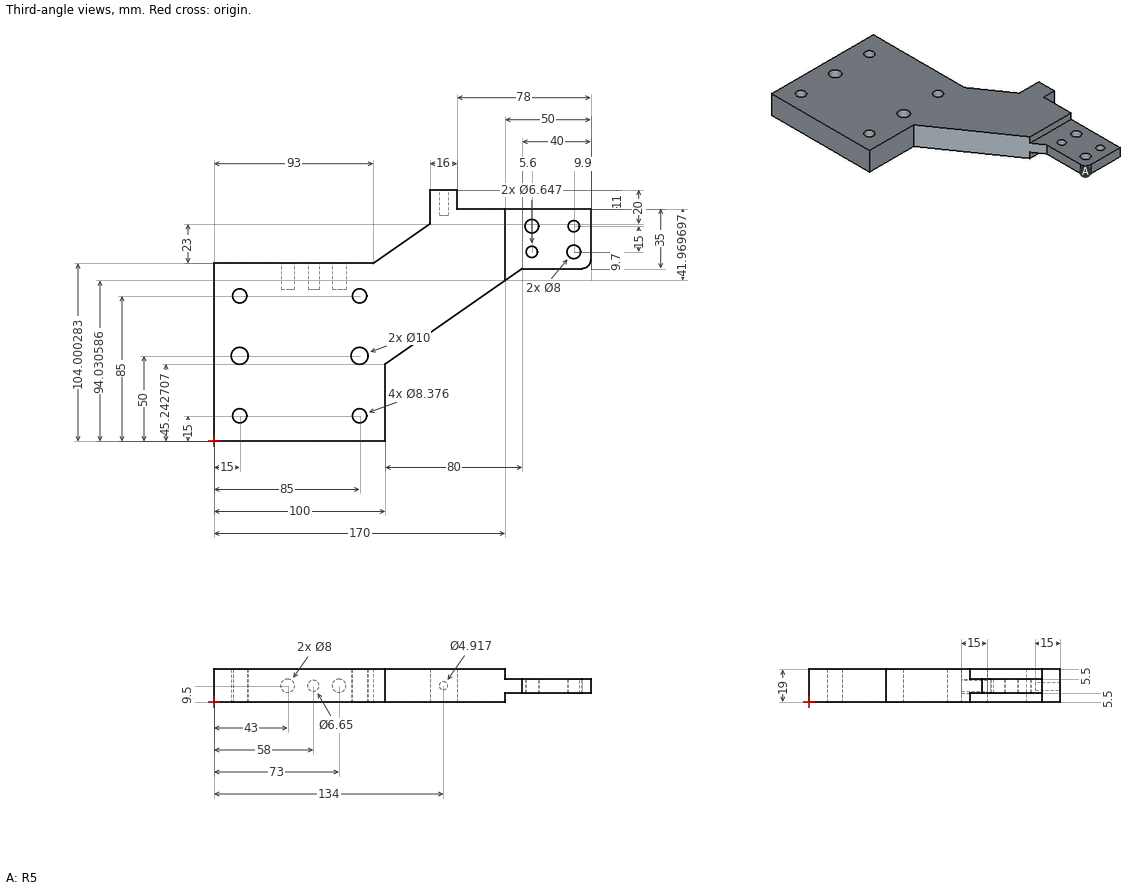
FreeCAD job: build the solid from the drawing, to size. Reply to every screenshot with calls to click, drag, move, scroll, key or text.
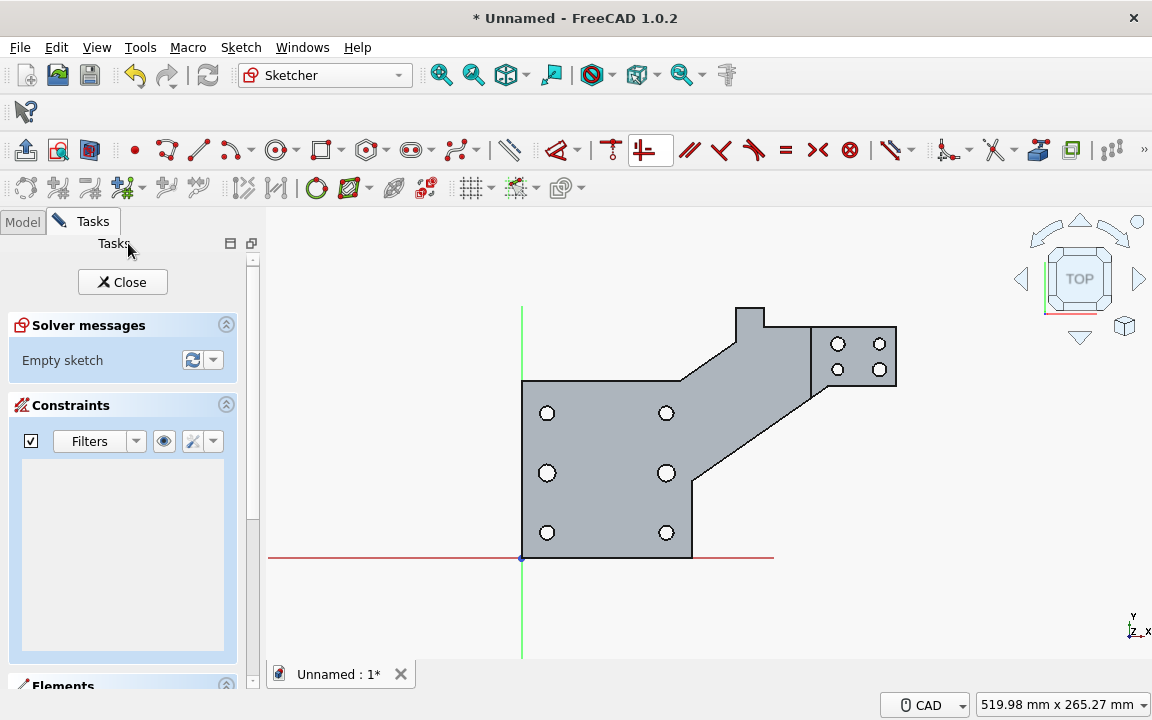
click(90, 150)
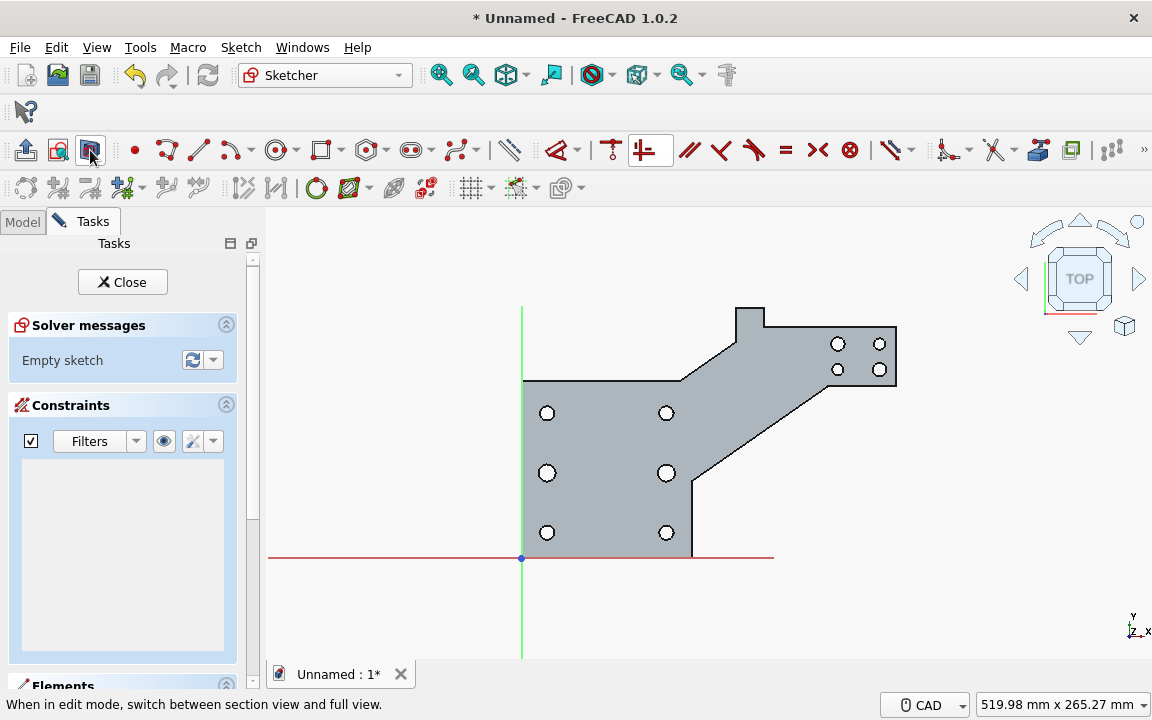
scroll(924, 339, up, 7)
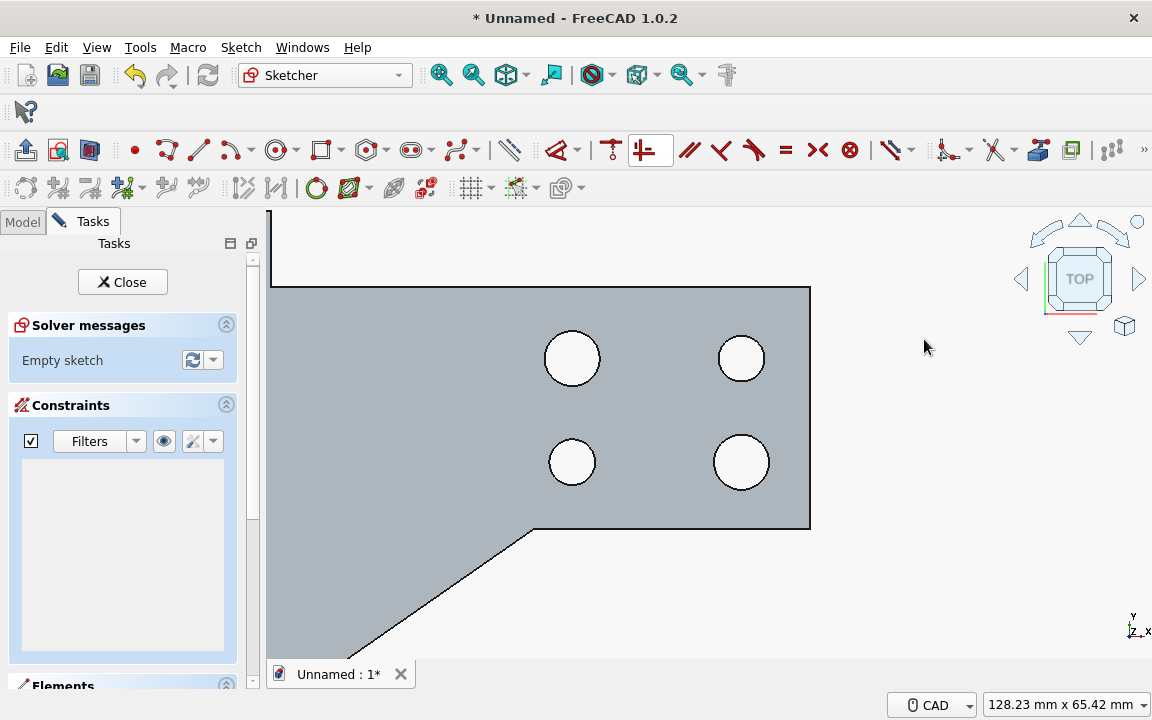
click(322, 150)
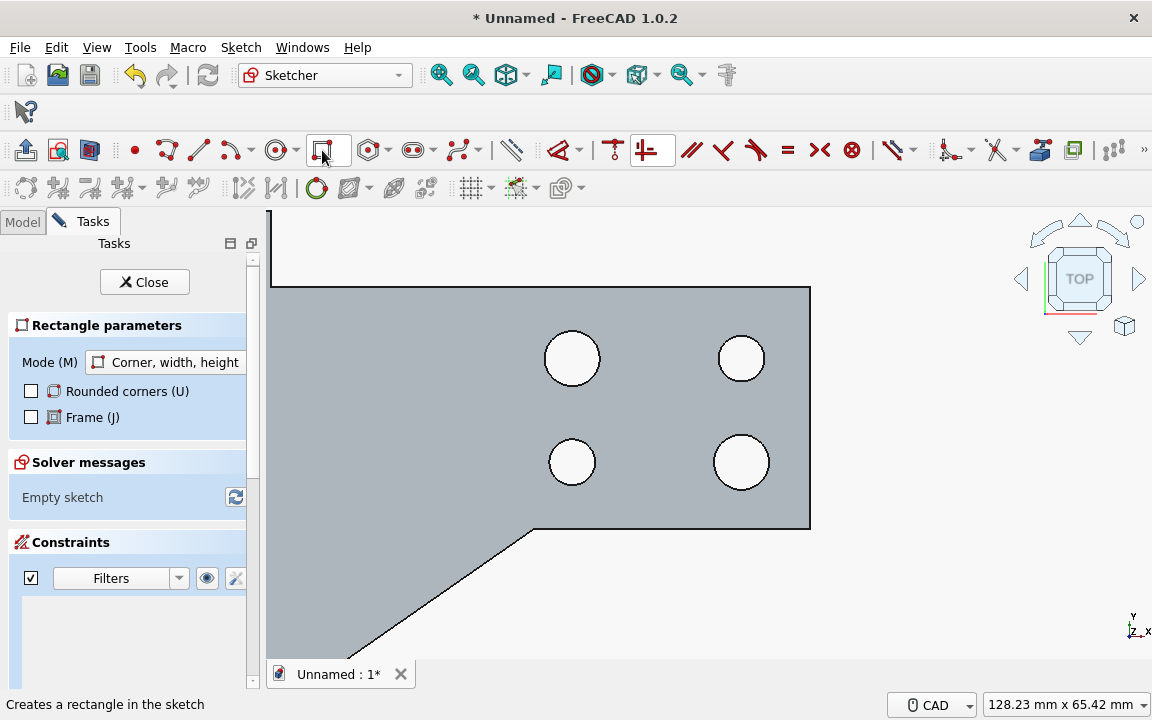
click(464, 287)
click(810, 577)
key(Escape)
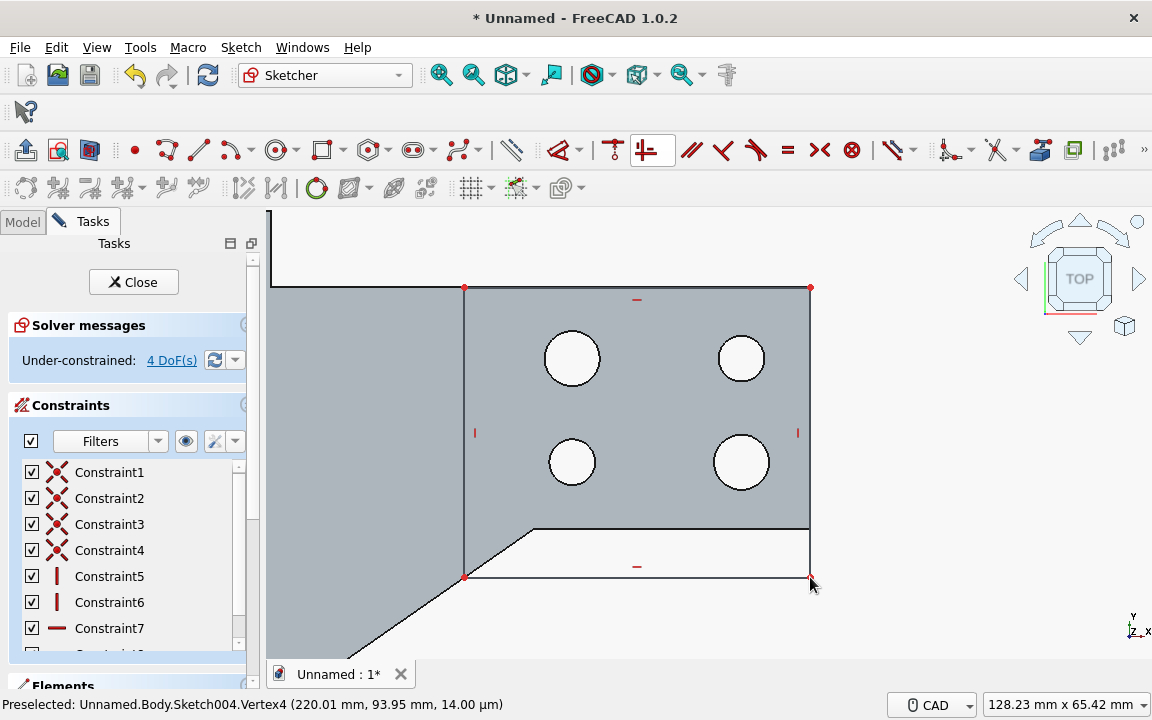
click(558, 150)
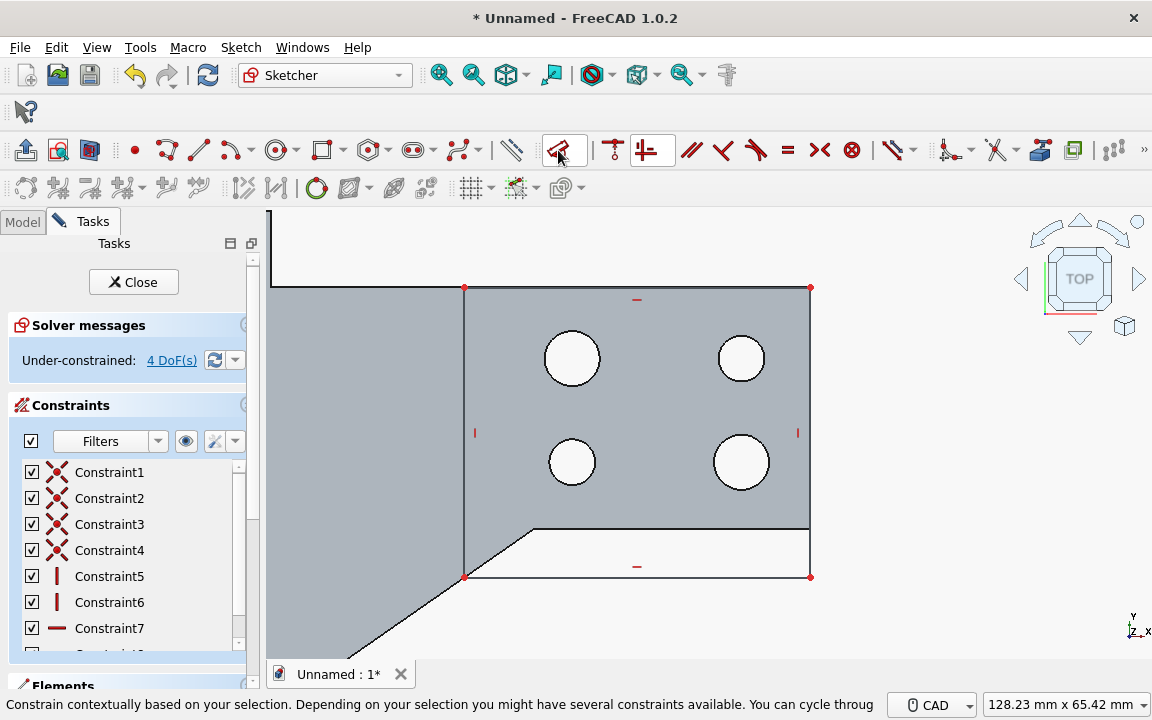
click(568, 578)
click(637, 612)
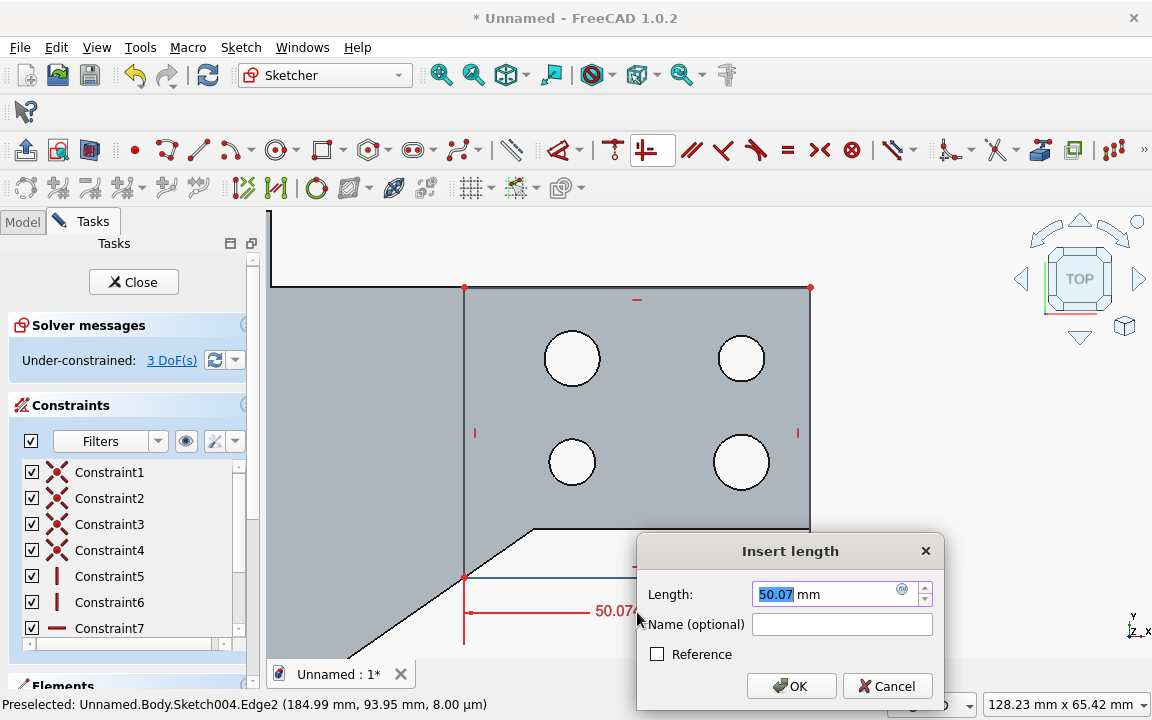
text(50)
key(Return)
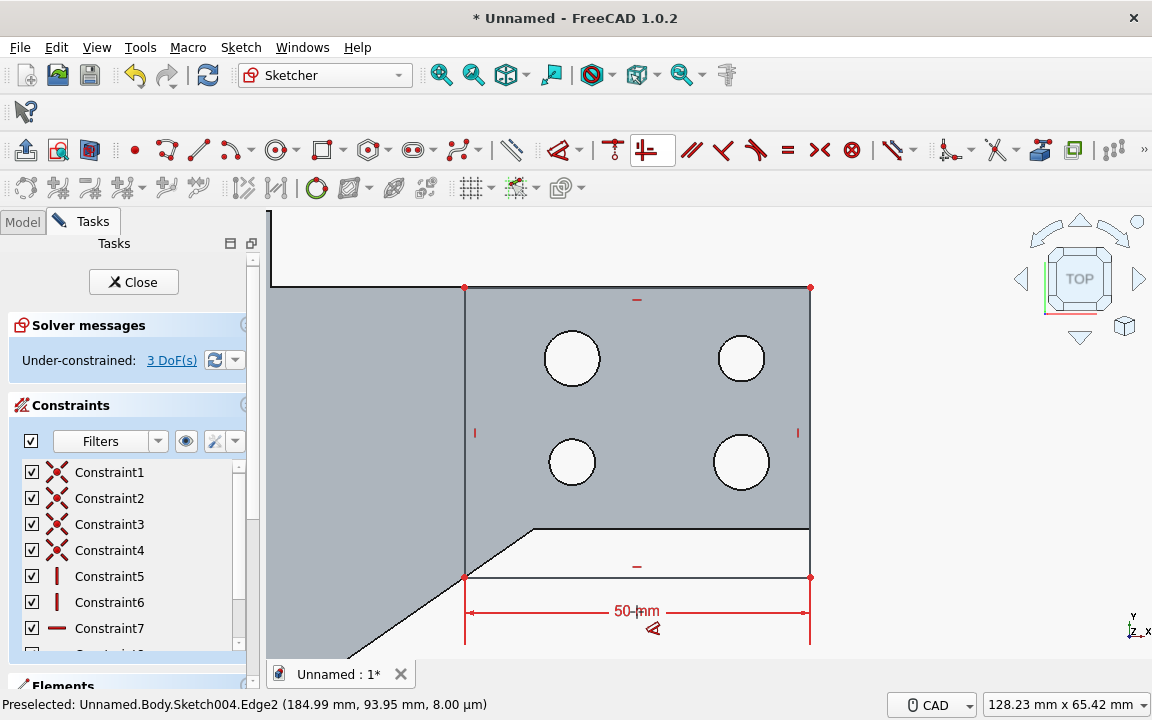
click(465, 288)
click(379, 254)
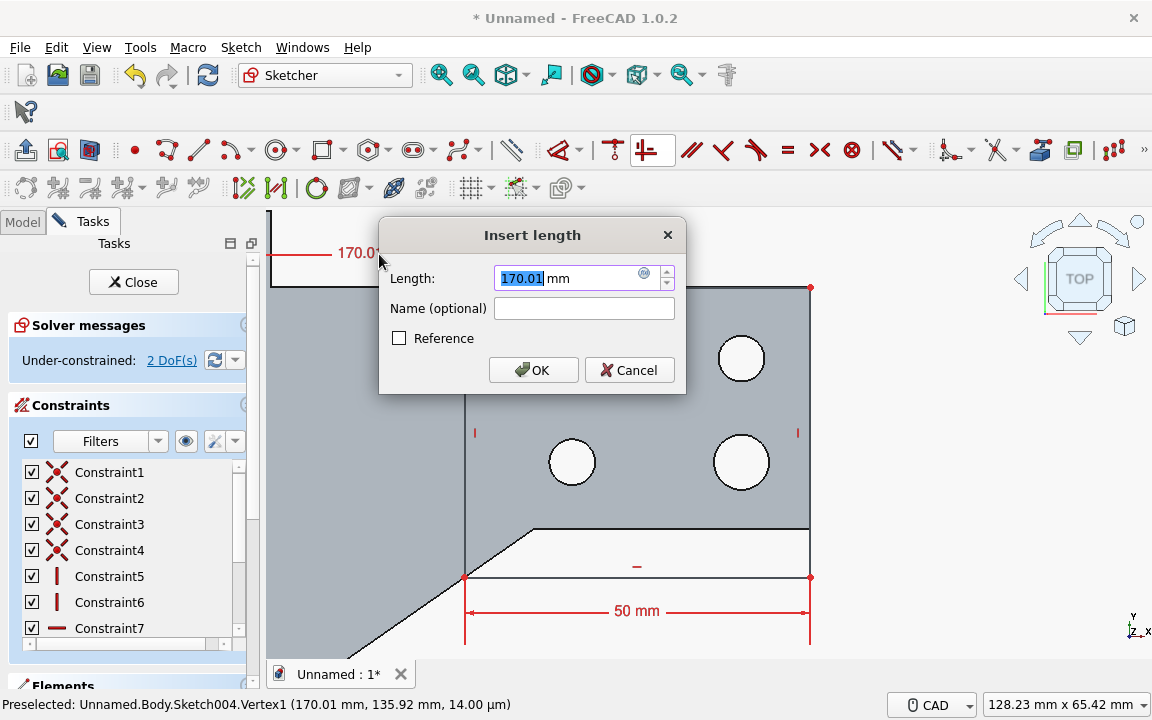
text(170)
key(Return)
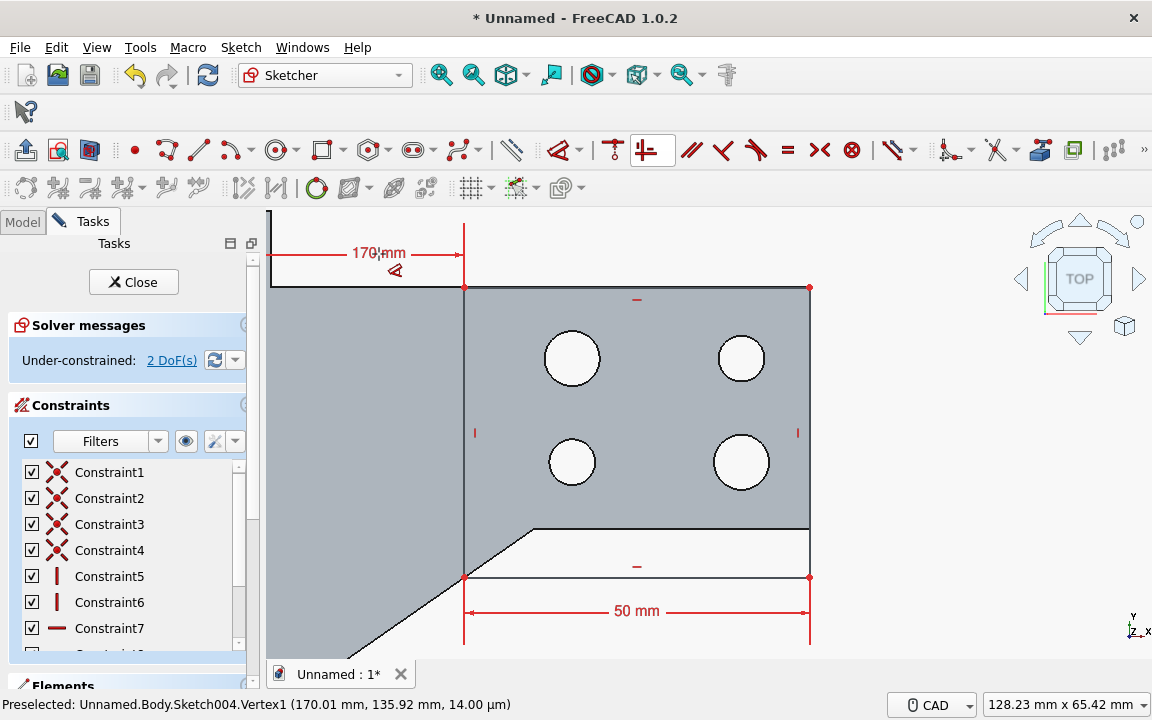
click(464, 375)
click(430, 433)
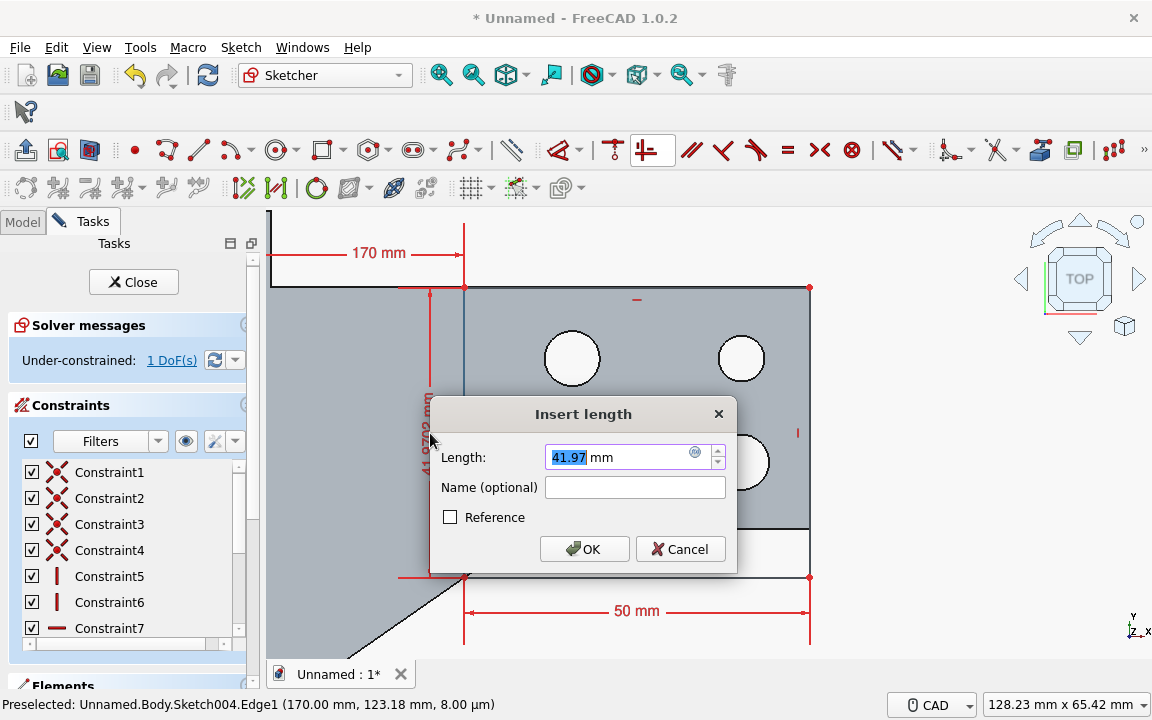
text(41.969697)
key(Return)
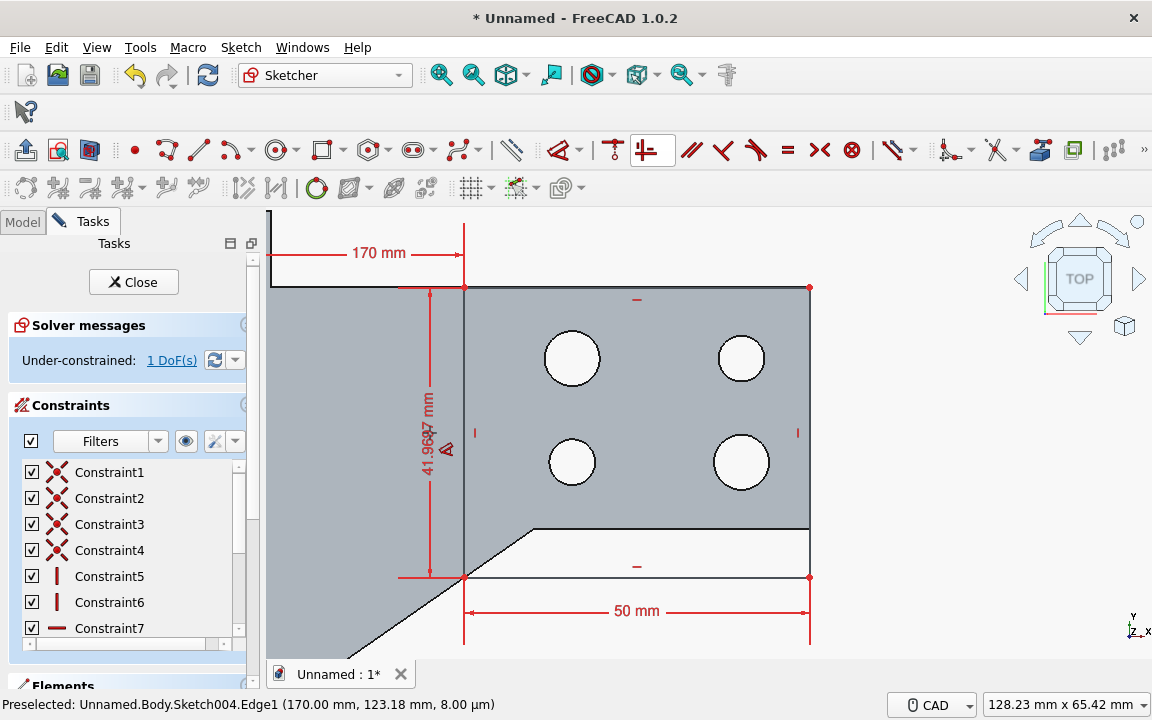
click(464, 578)
click(498, 604)